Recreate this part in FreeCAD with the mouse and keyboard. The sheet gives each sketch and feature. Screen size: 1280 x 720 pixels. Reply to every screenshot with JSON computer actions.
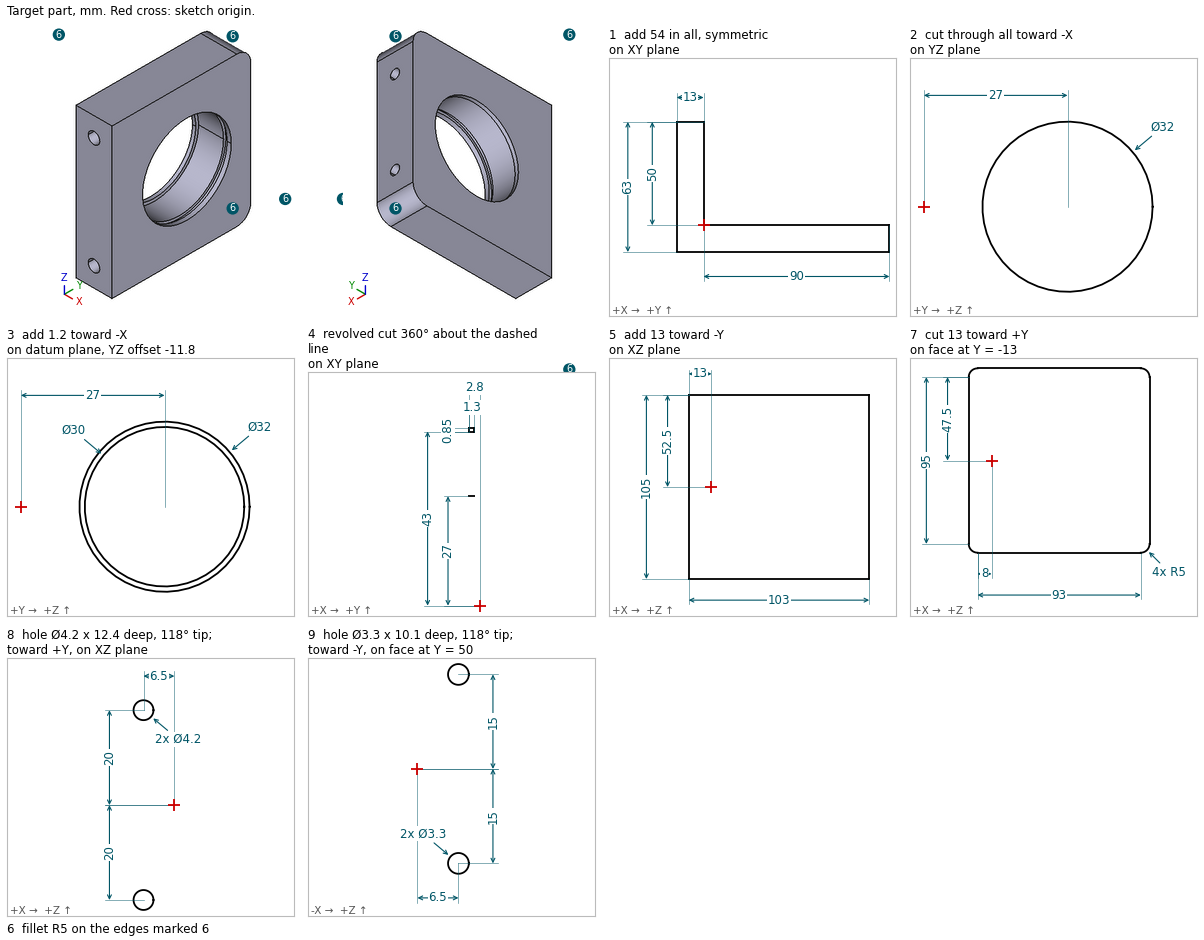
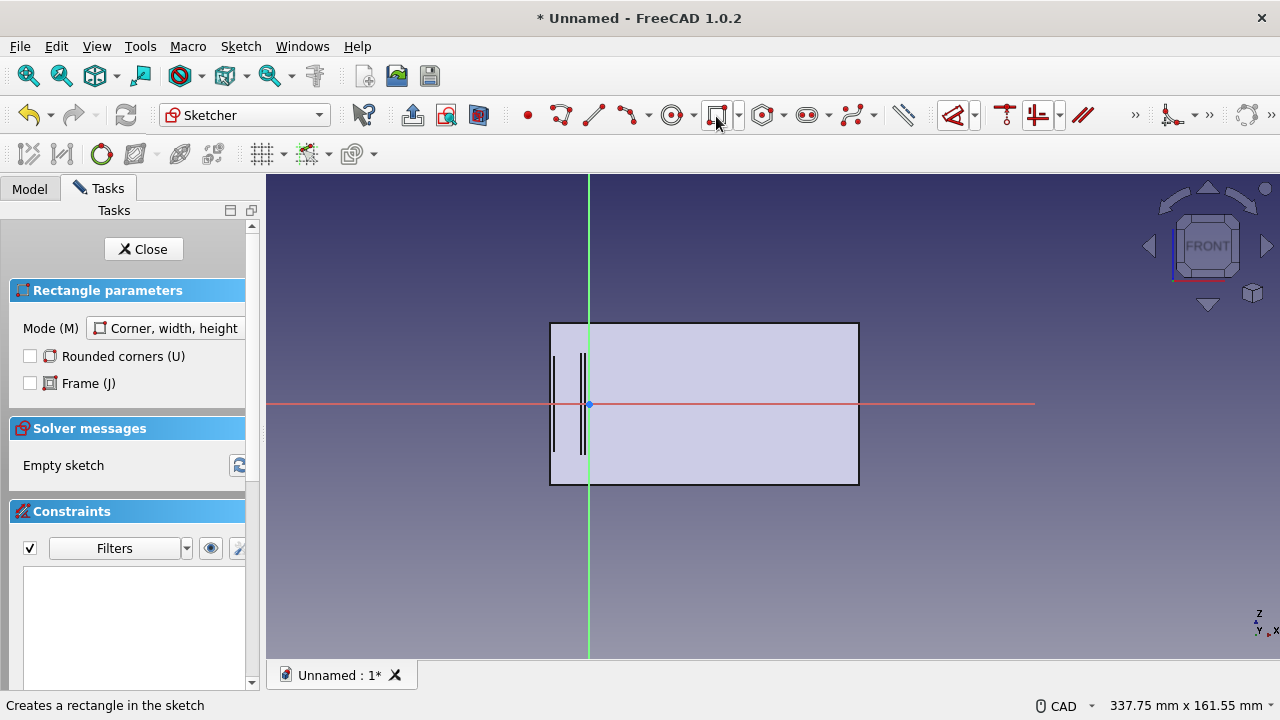
{"action": "left_click", "coordinate": [550, 247]}
{"action": "left_click", "coordinate": [859, 562]}
{"action": "key", "text": "Escape"}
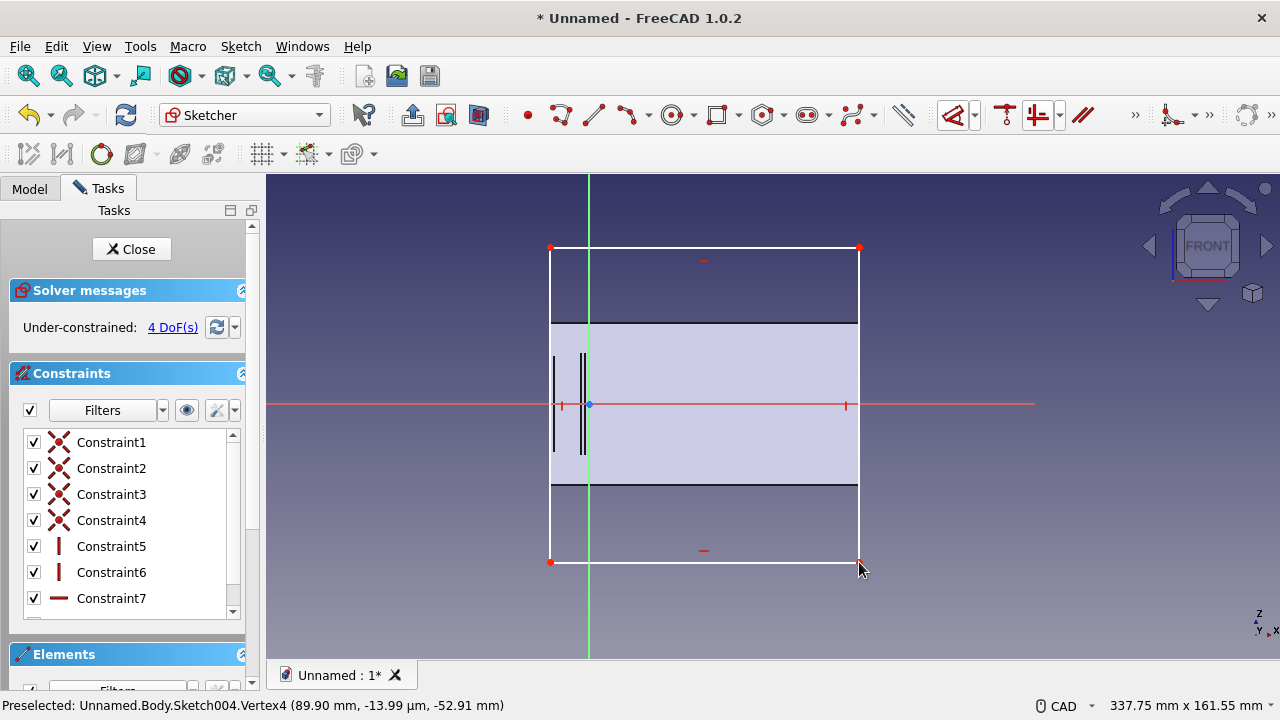
{"action": "left_click", "coordinate": [550, 343]}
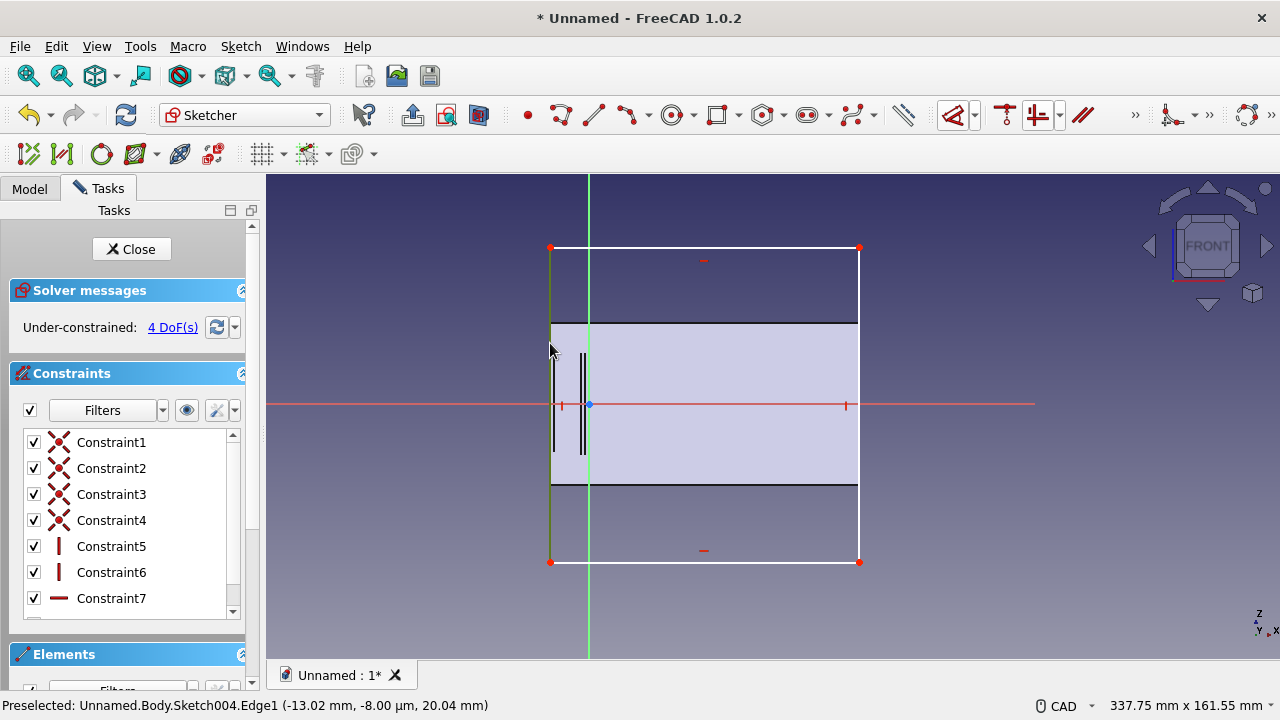
{"action": "key", "text": "i"}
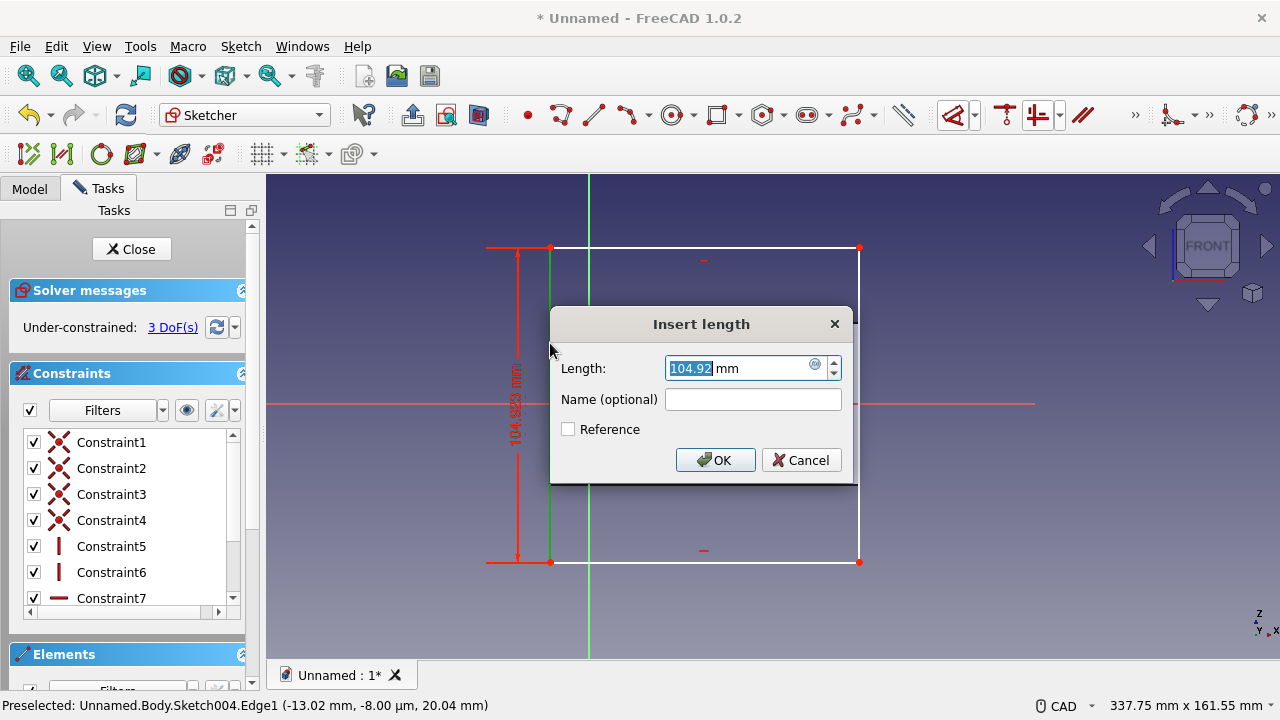
{"action": "type", "text": "105"}
{"action": "key", "text": "Return"}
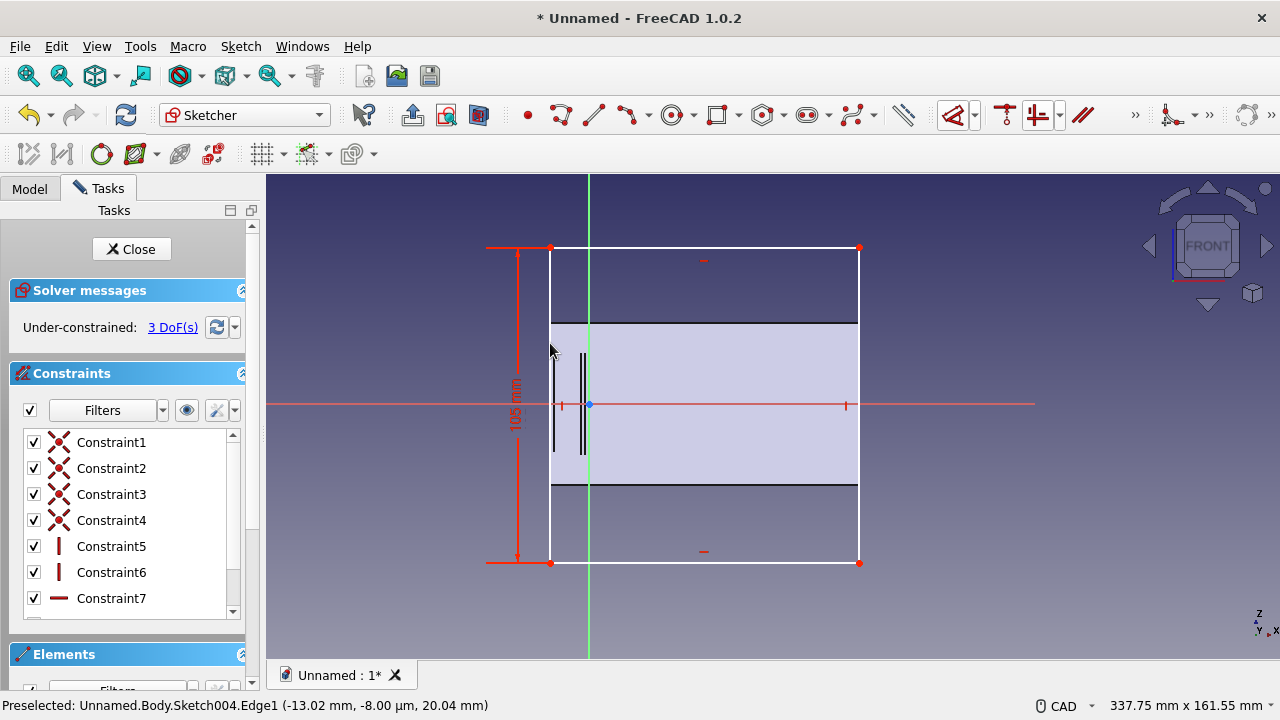
{"action": "left_click", "coordinate": [643, 563]}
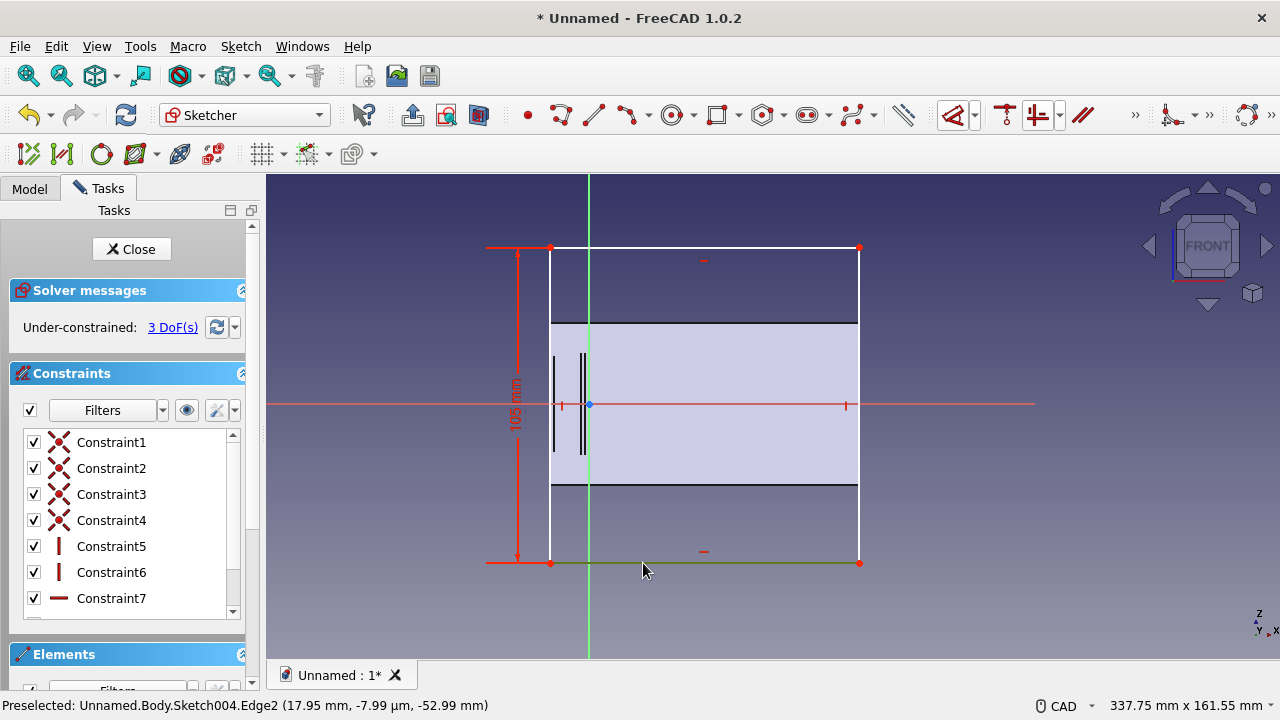
{"action": "key", "text": "l"}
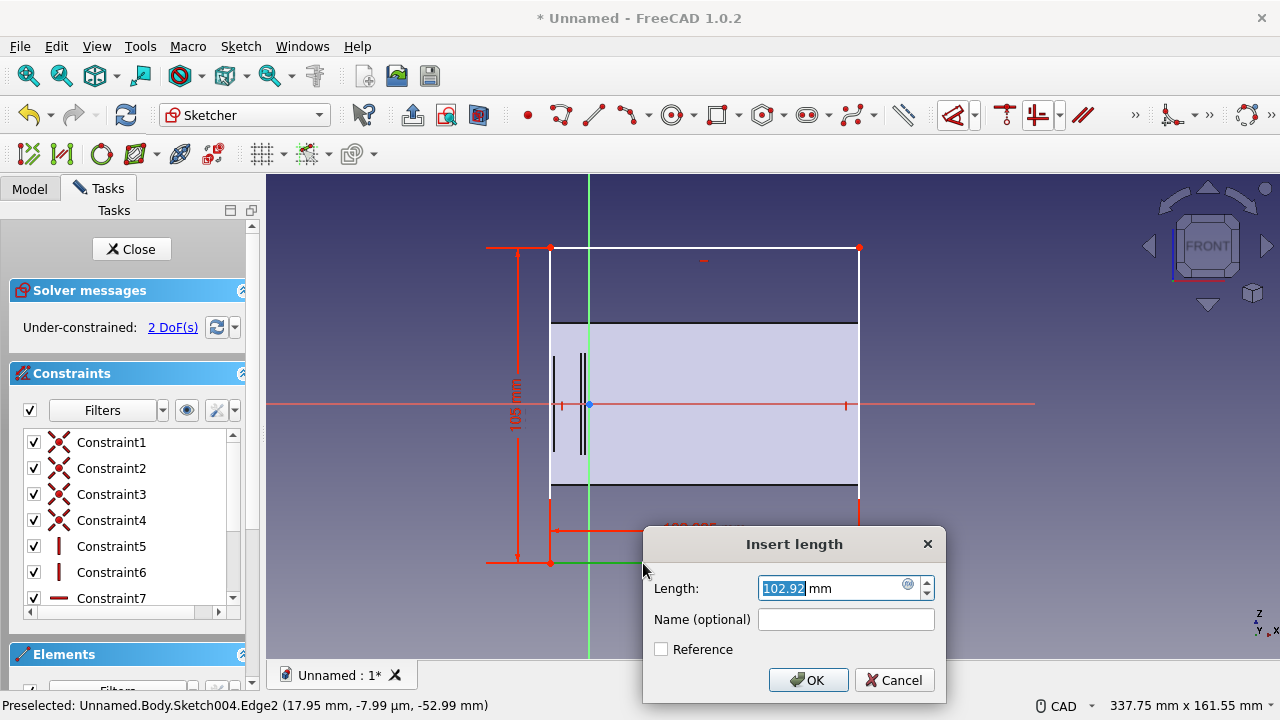
{"action": "type", "text": "103"}
{"action": "key", "text": "Return"}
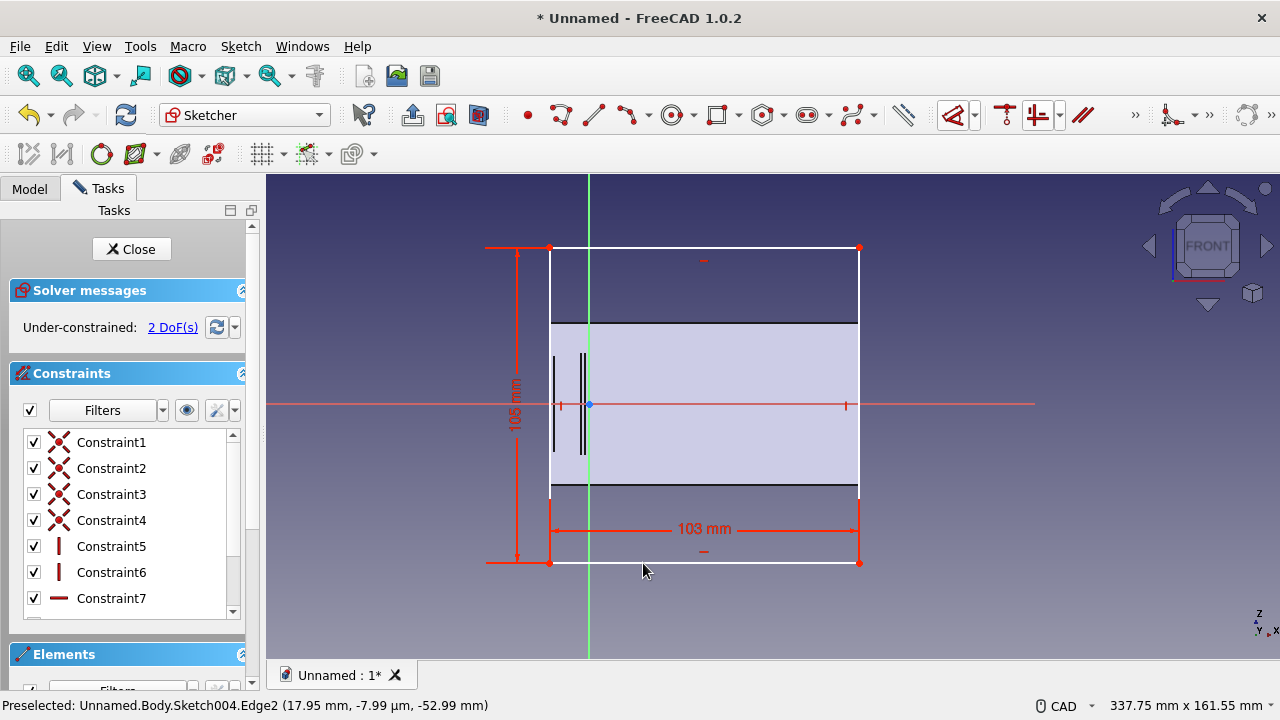
{"action": "left_click", "coordinate": [550, 248]}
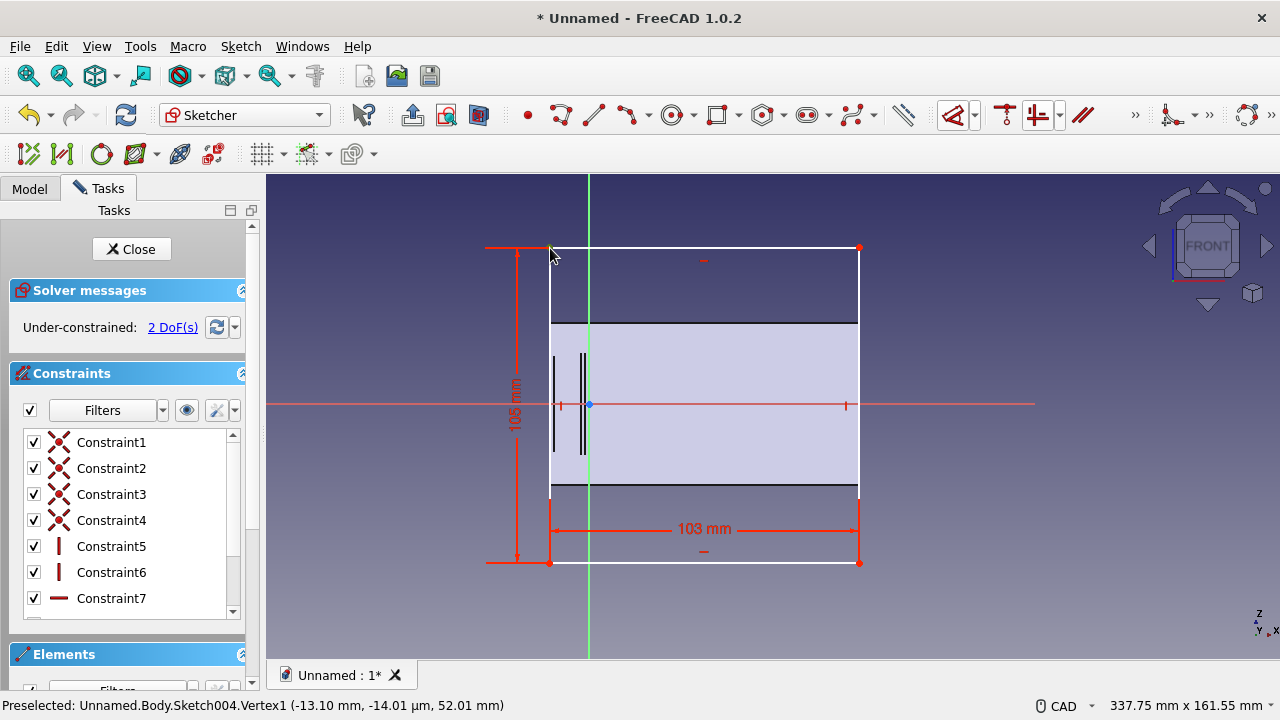
{"action": "left_click", "coordinate": [974, 116]}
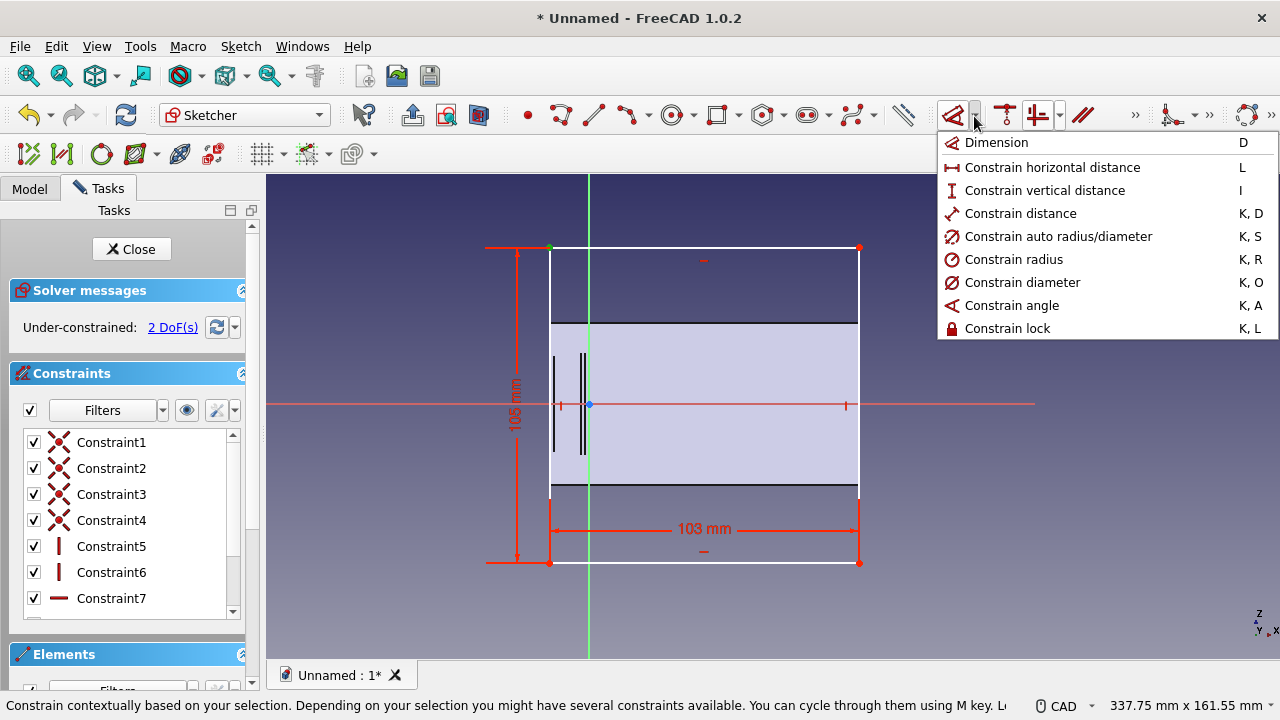
{"action": "left_click", "coordinate": [1108, 168]}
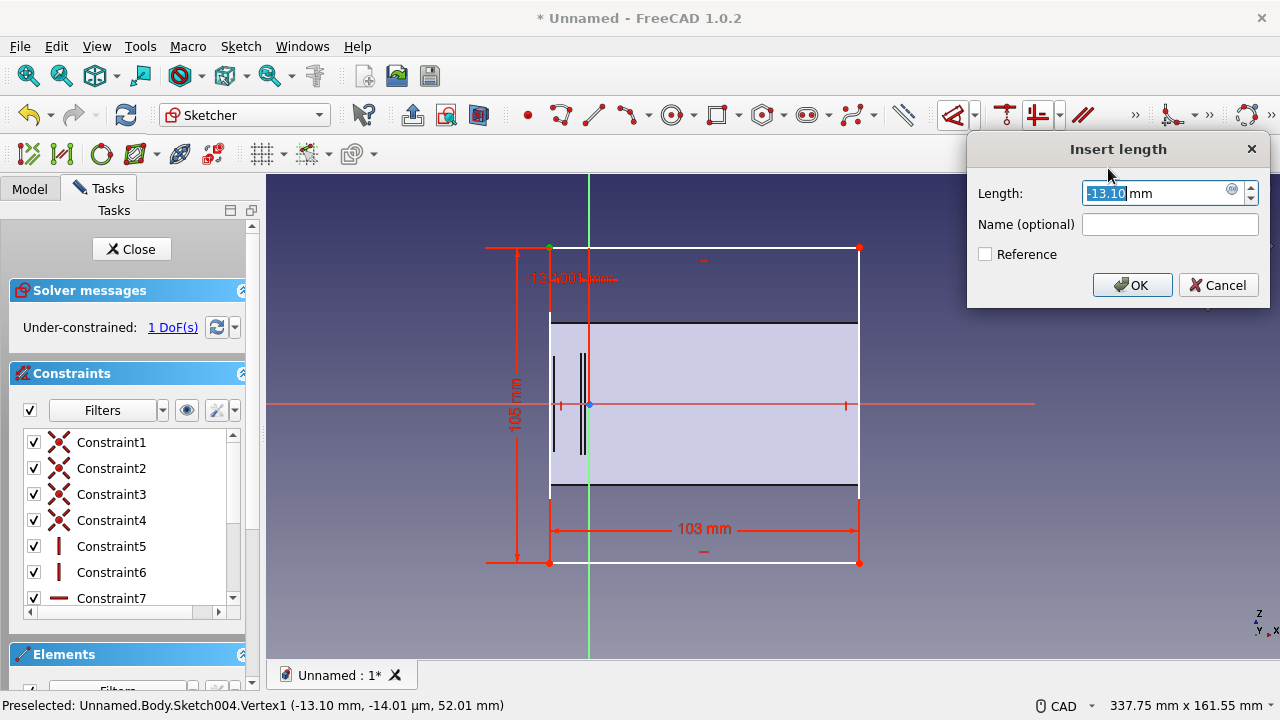
{"action": "type", "text": "-13"}
{"action": "key", "text": "Return"}